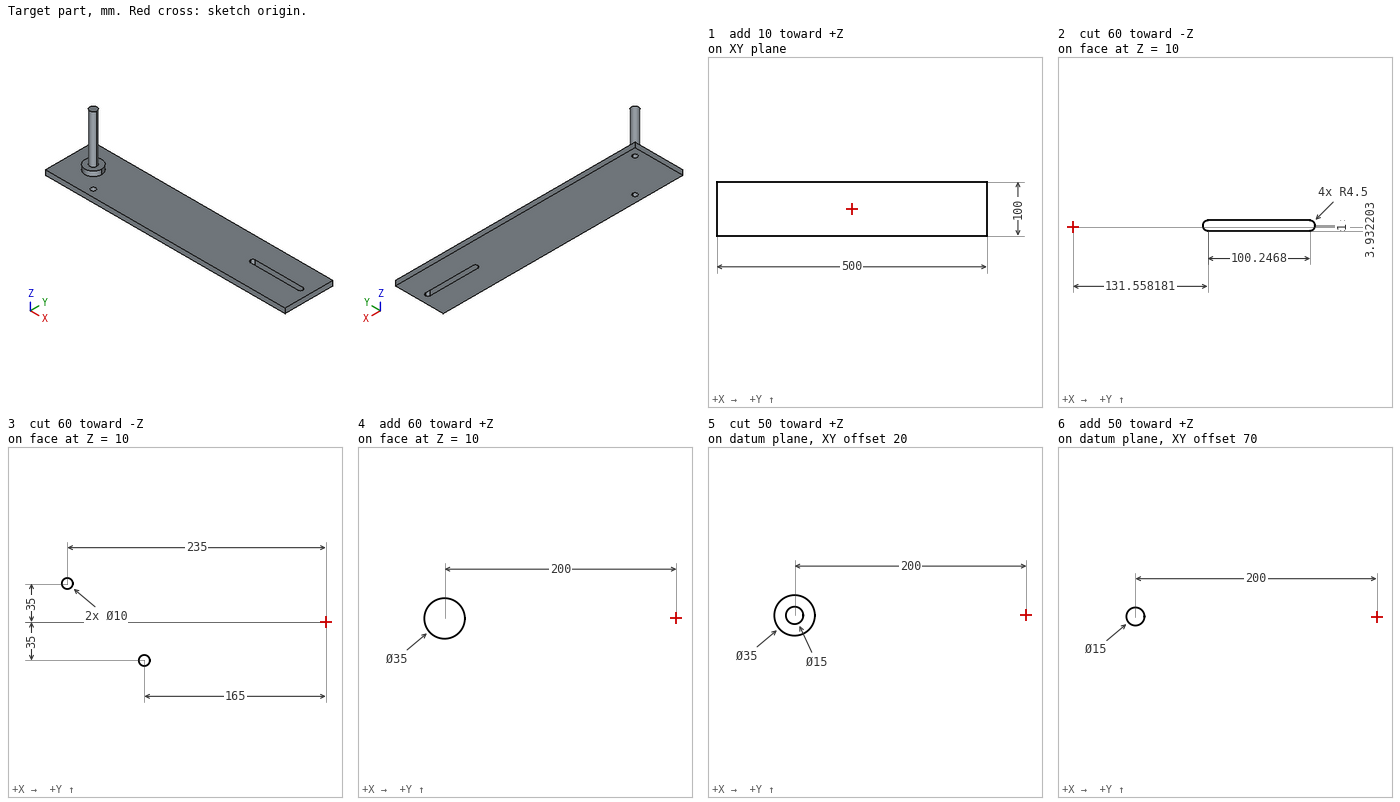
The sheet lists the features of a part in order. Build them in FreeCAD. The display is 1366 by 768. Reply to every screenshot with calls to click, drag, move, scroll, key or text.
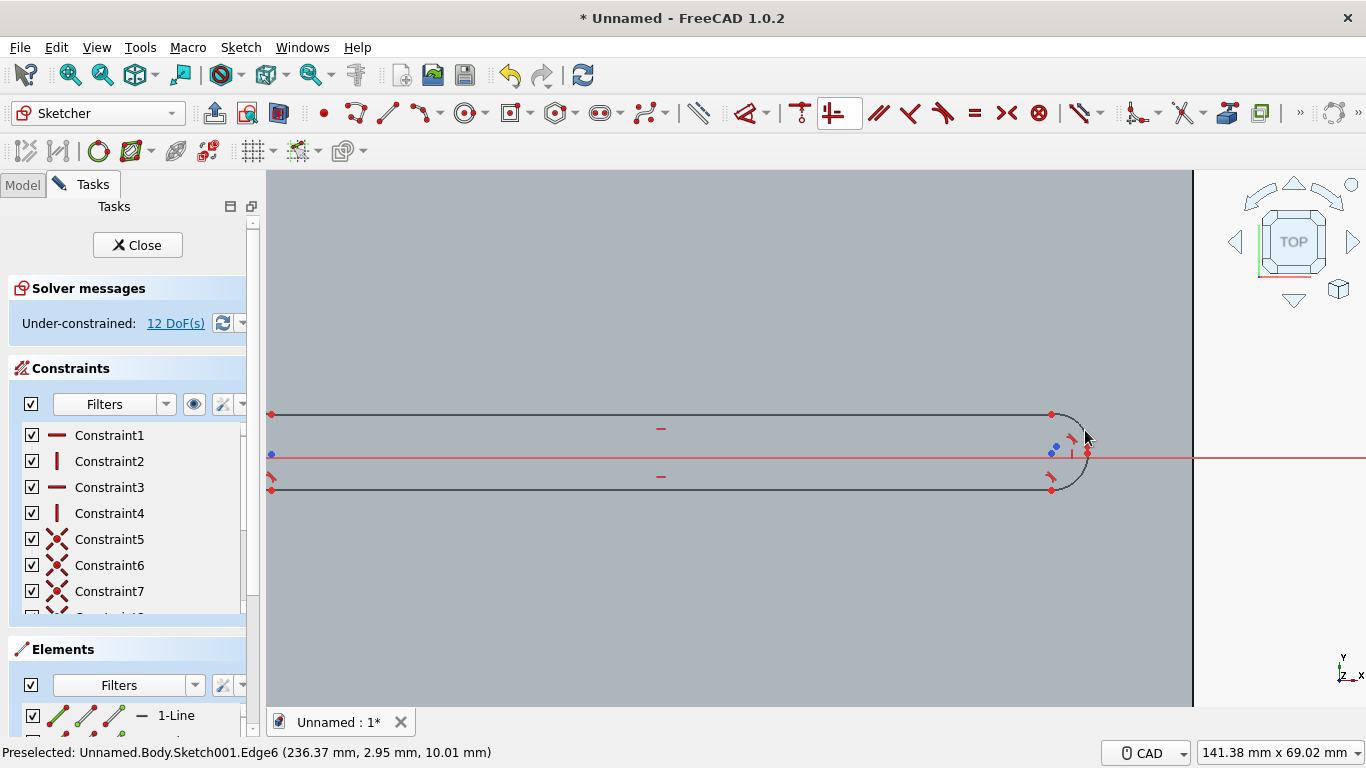
click(818, 415)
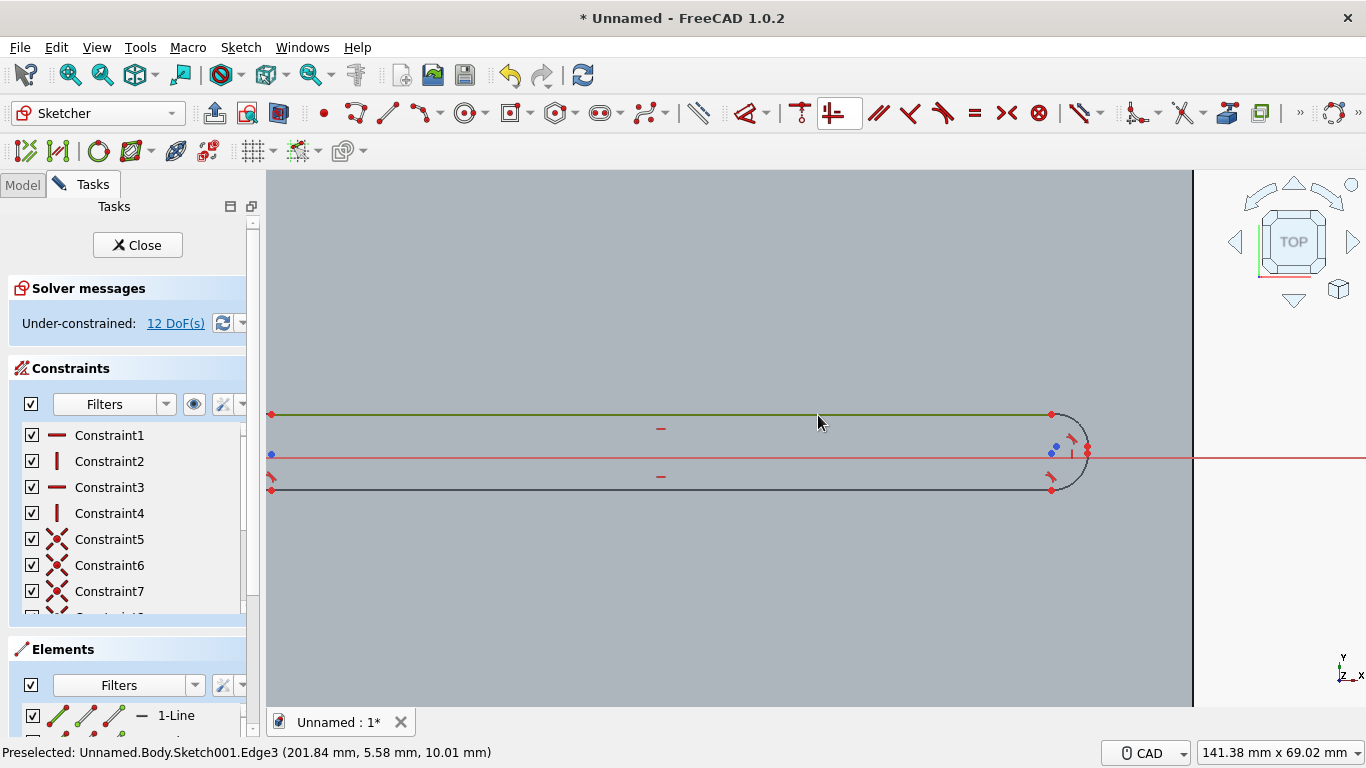
click(1084, 430)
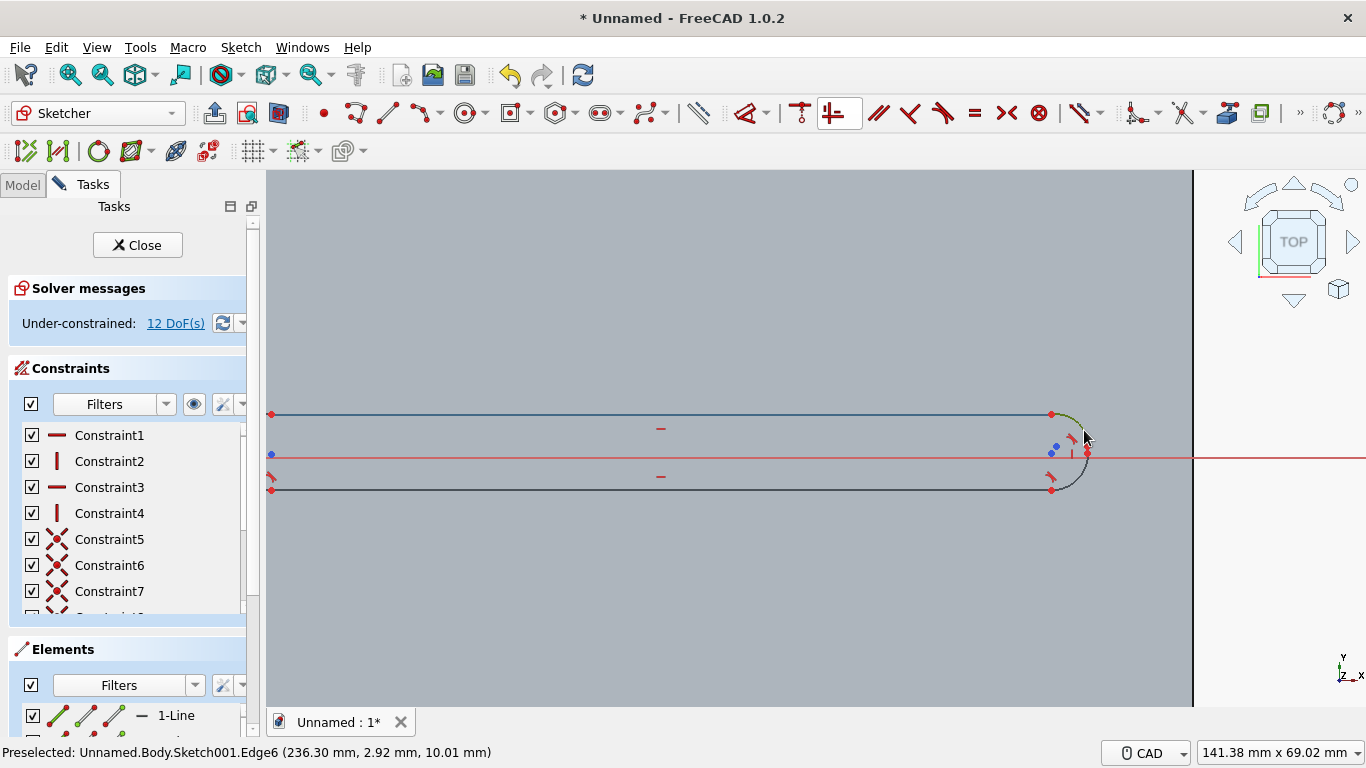
click(944, 114)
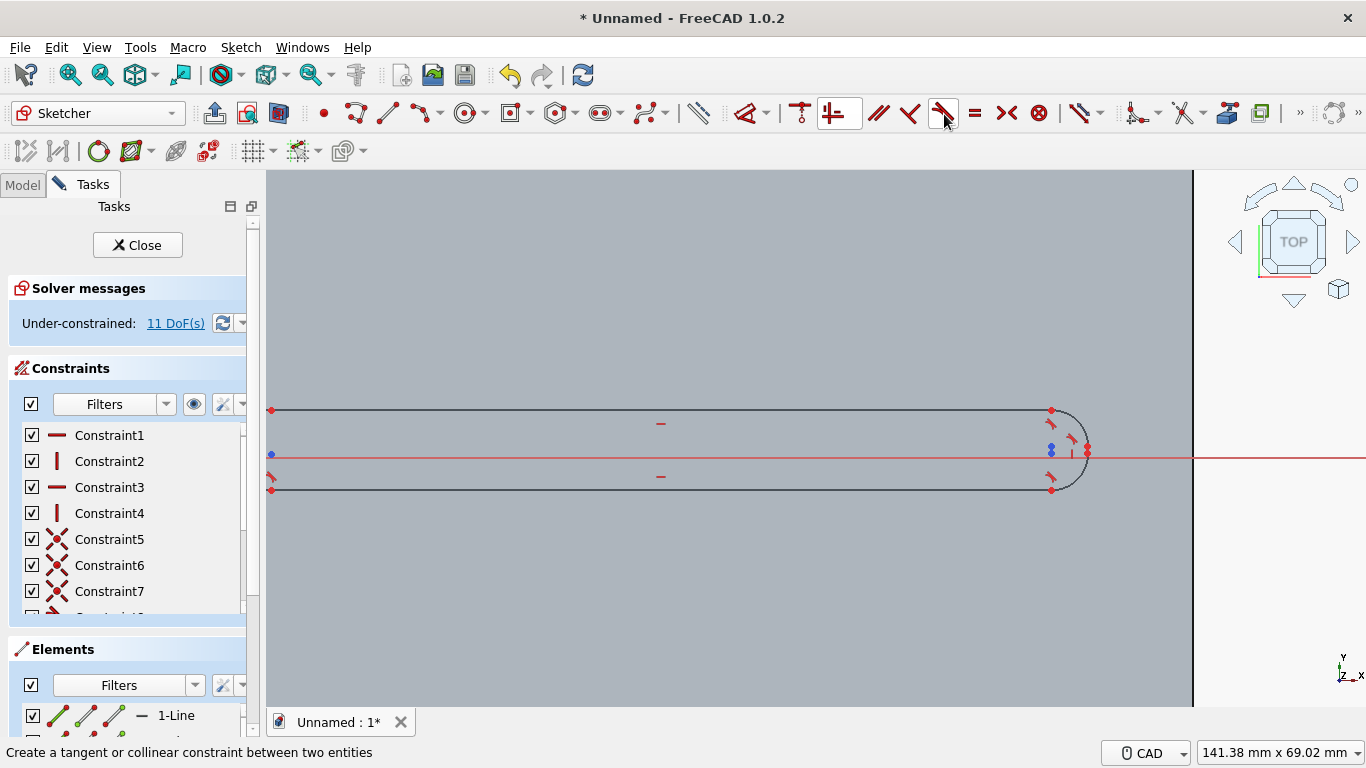
click(818, 410)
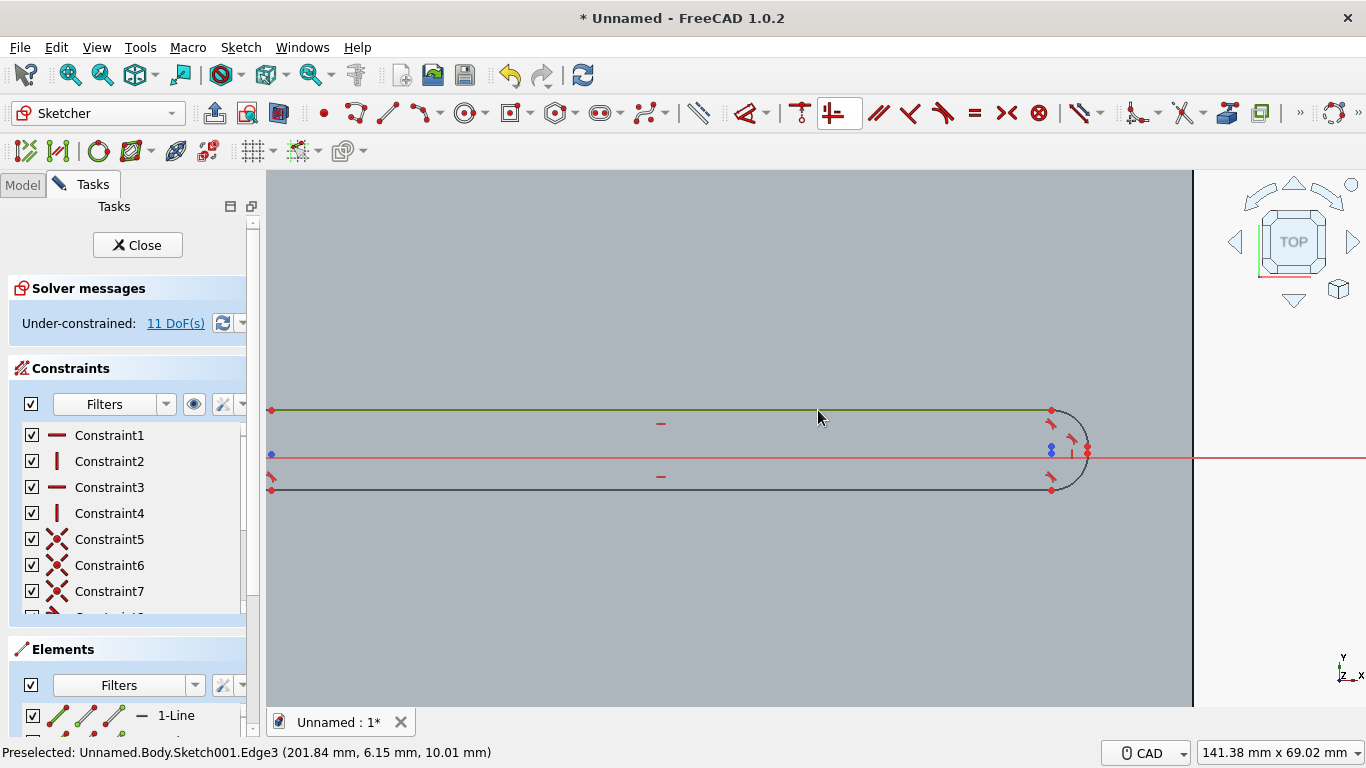
scroll(1085, 432, down, 5)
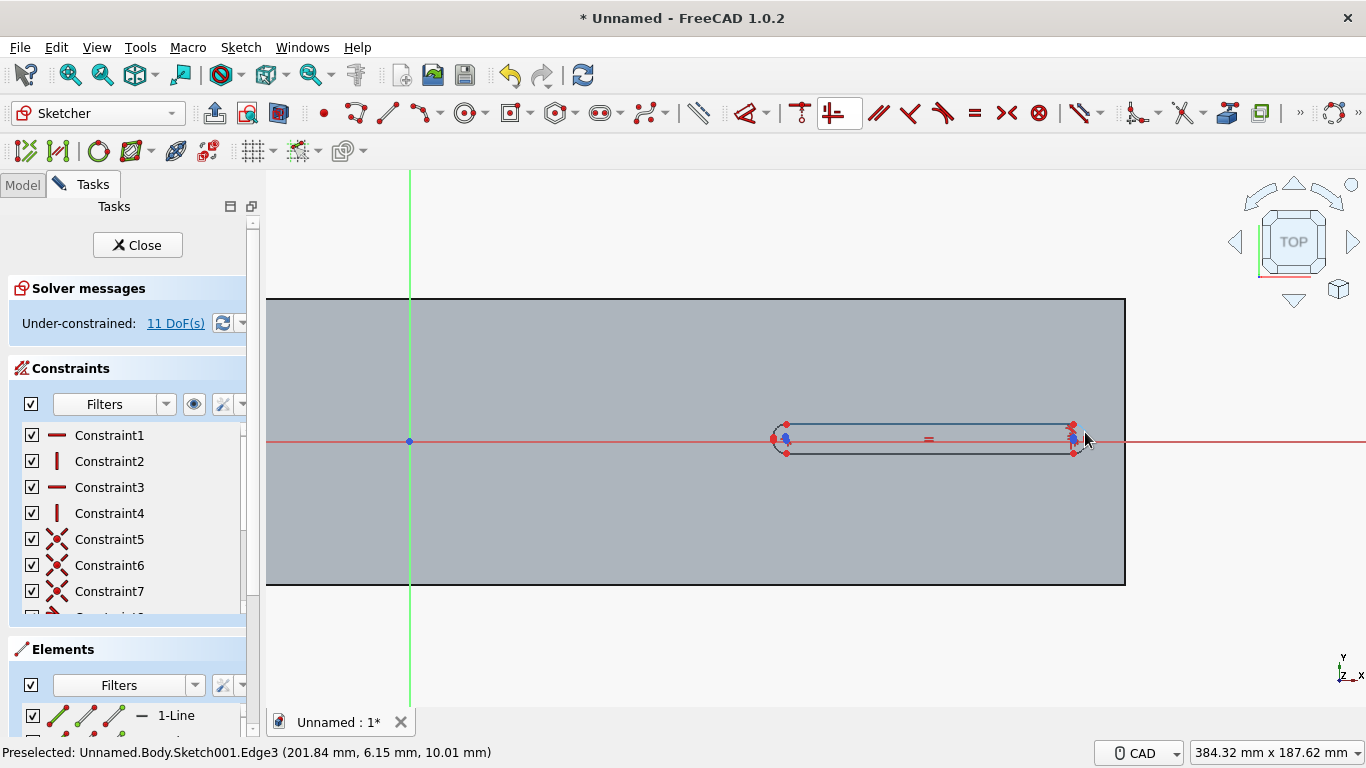
scroll(780, 426, up, 4)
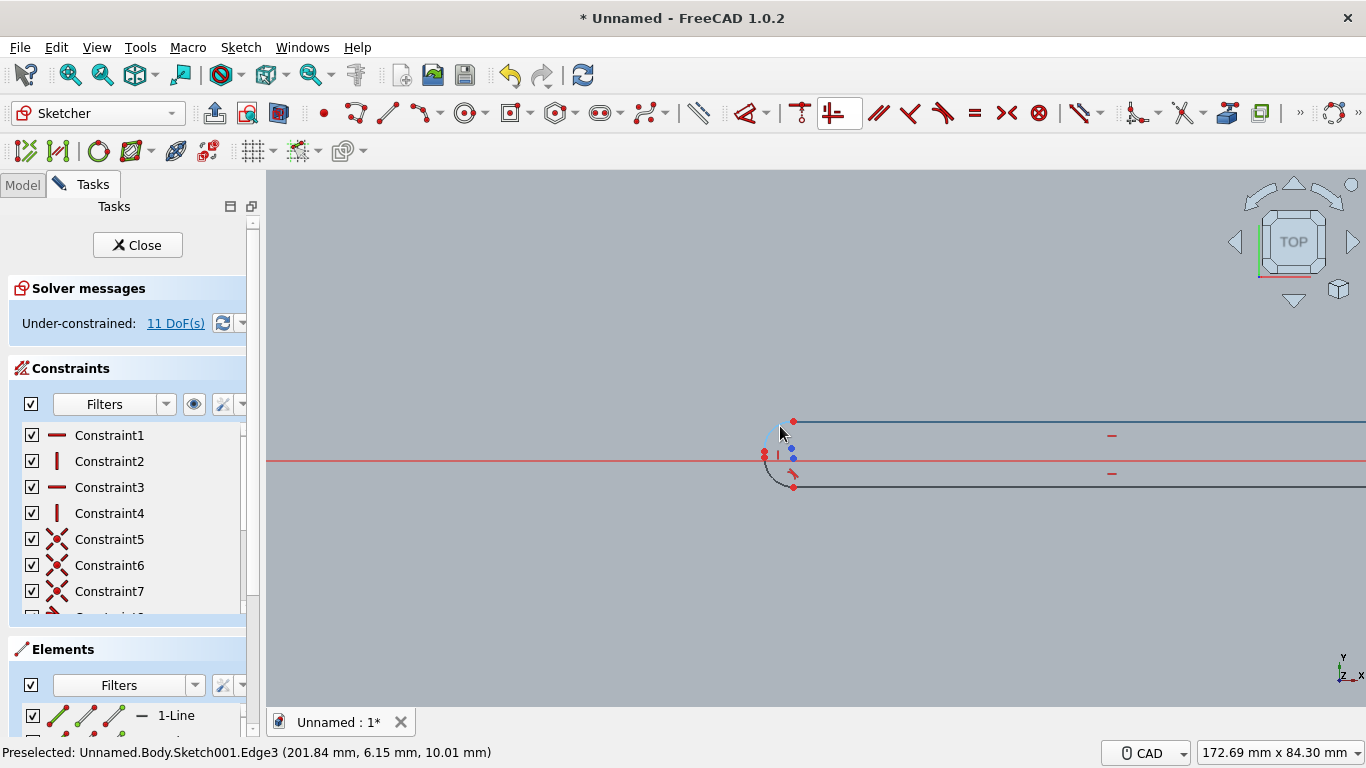
click(780, 424)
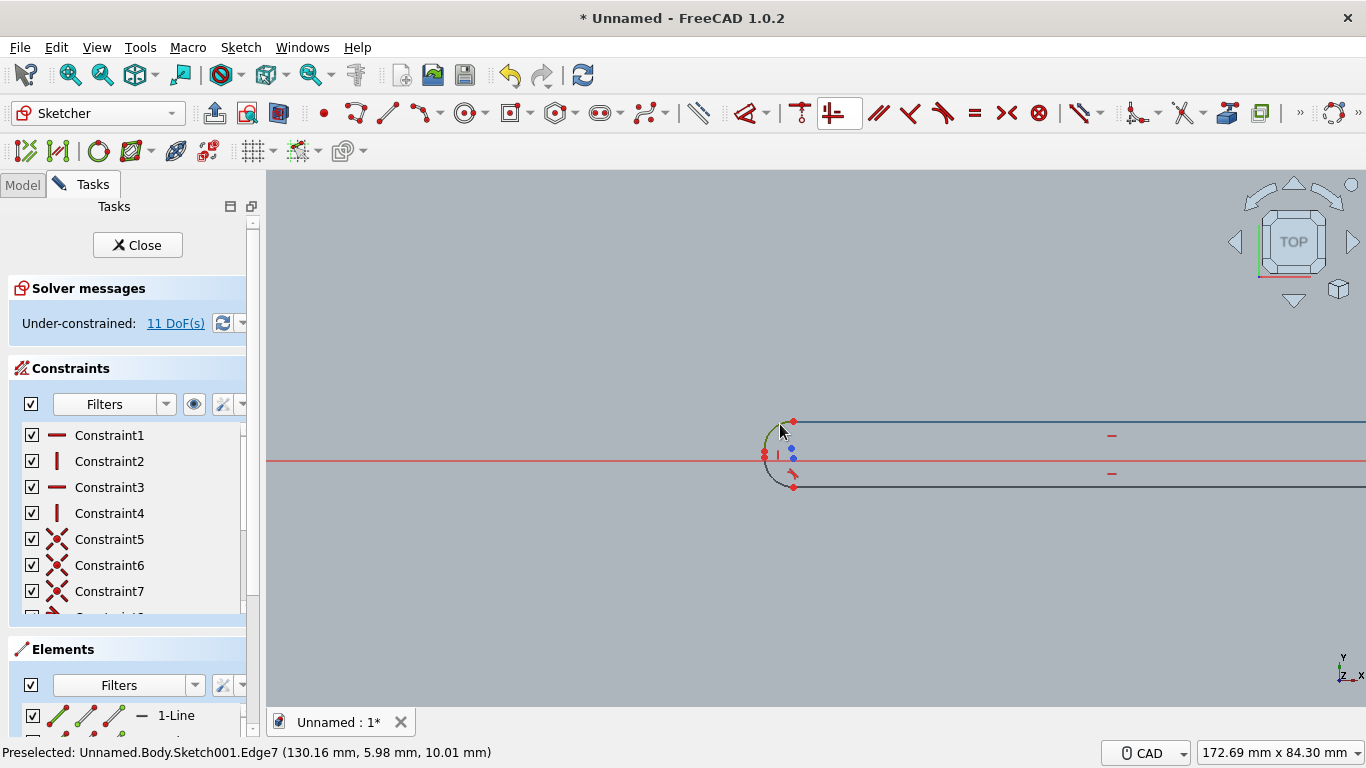
click(944, 114)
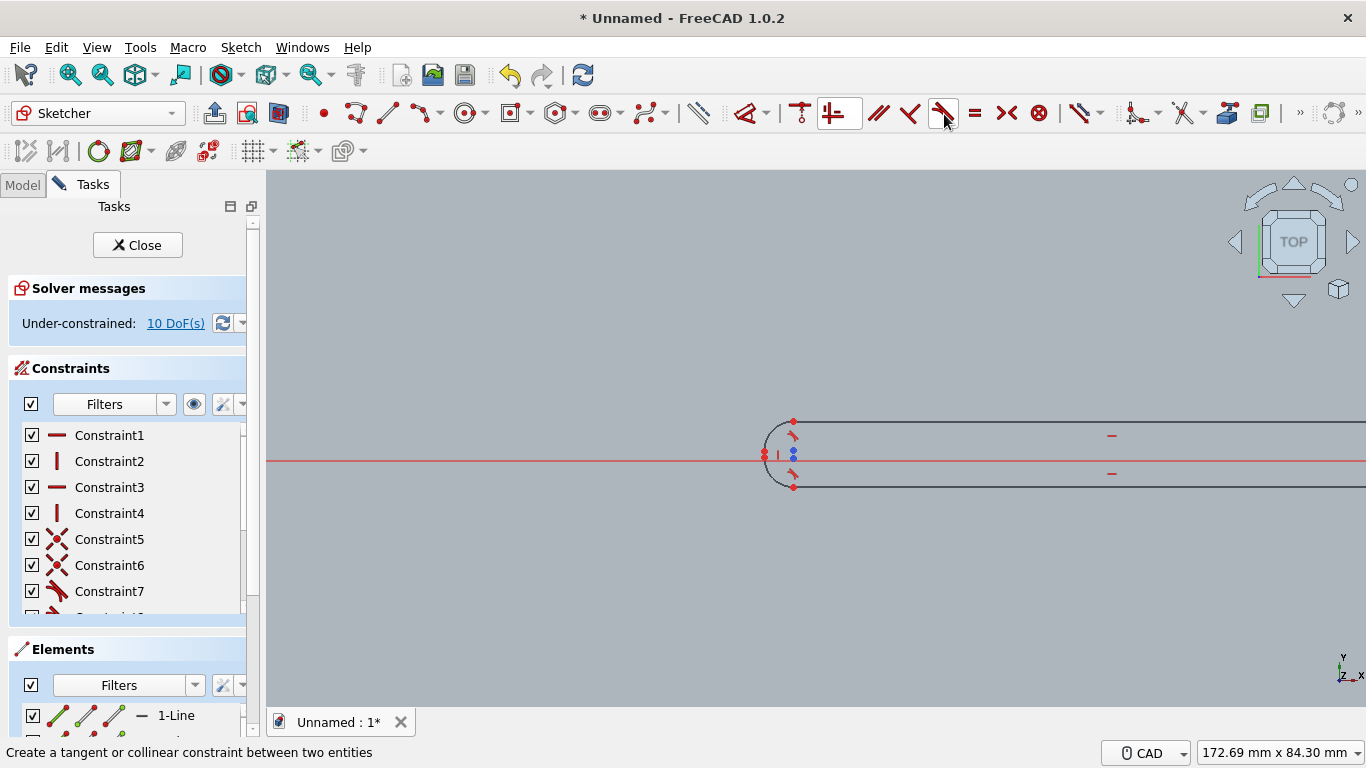
scroll(765, 454, up, 8)